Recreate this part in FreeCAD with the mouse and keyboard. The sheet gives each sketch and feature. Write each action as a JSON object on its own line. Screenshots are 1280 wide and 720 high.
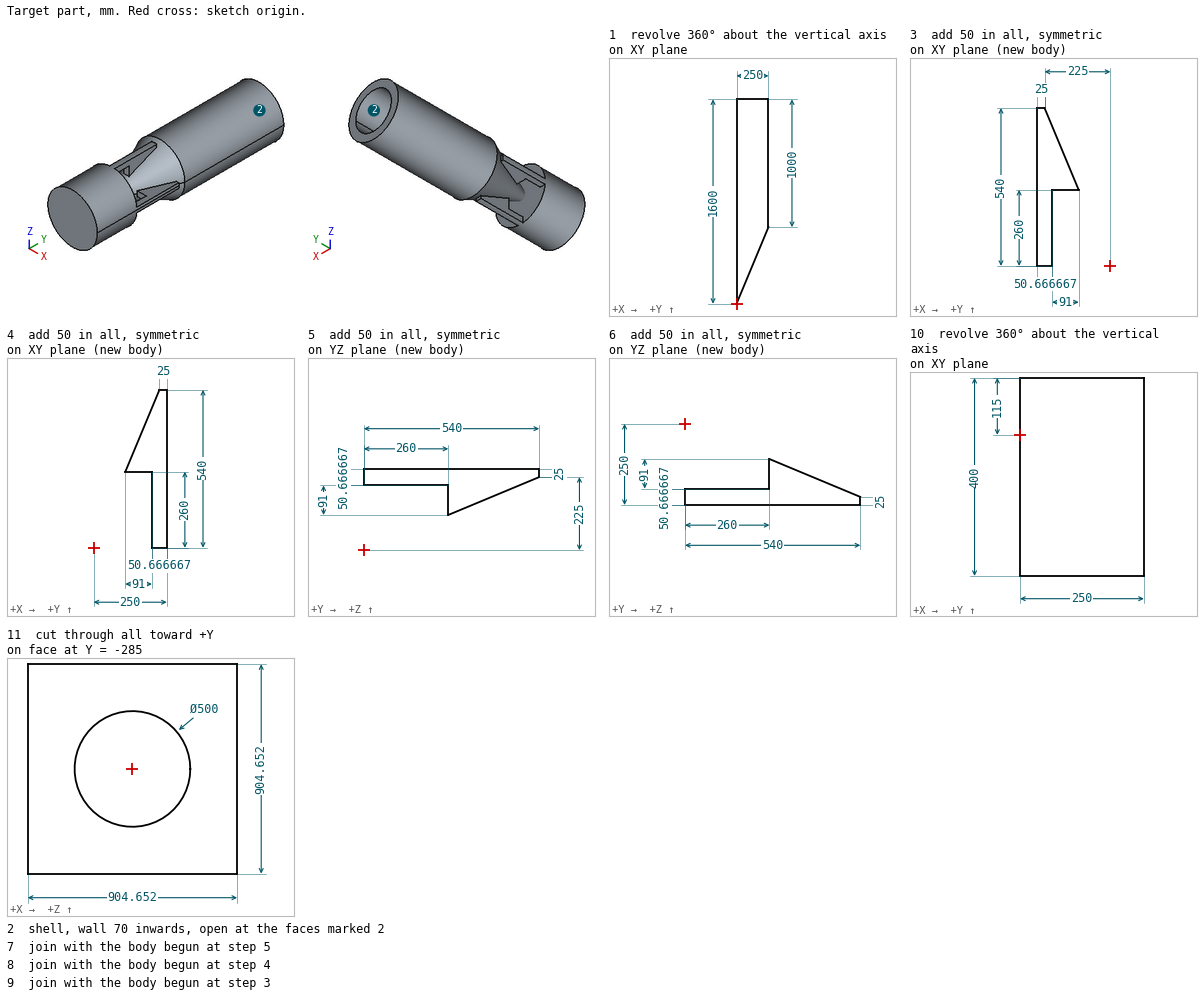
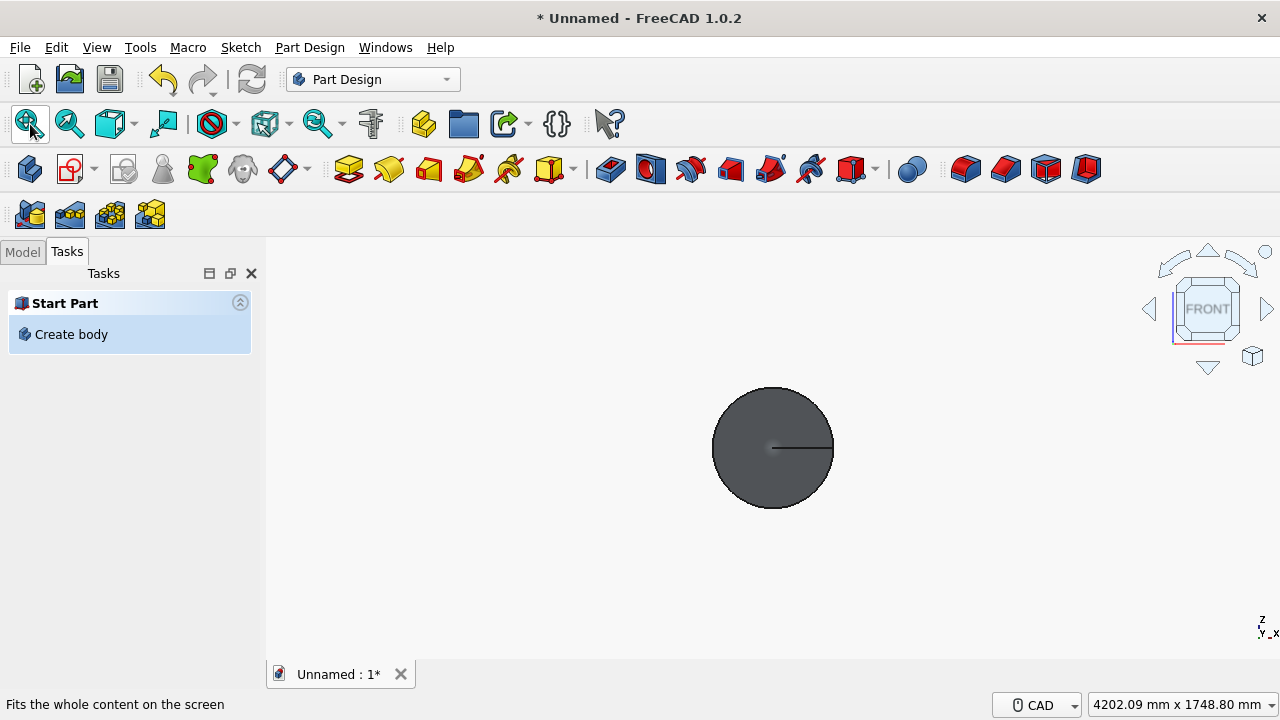
{"action": "left_click", "coordinate": [30, 124]}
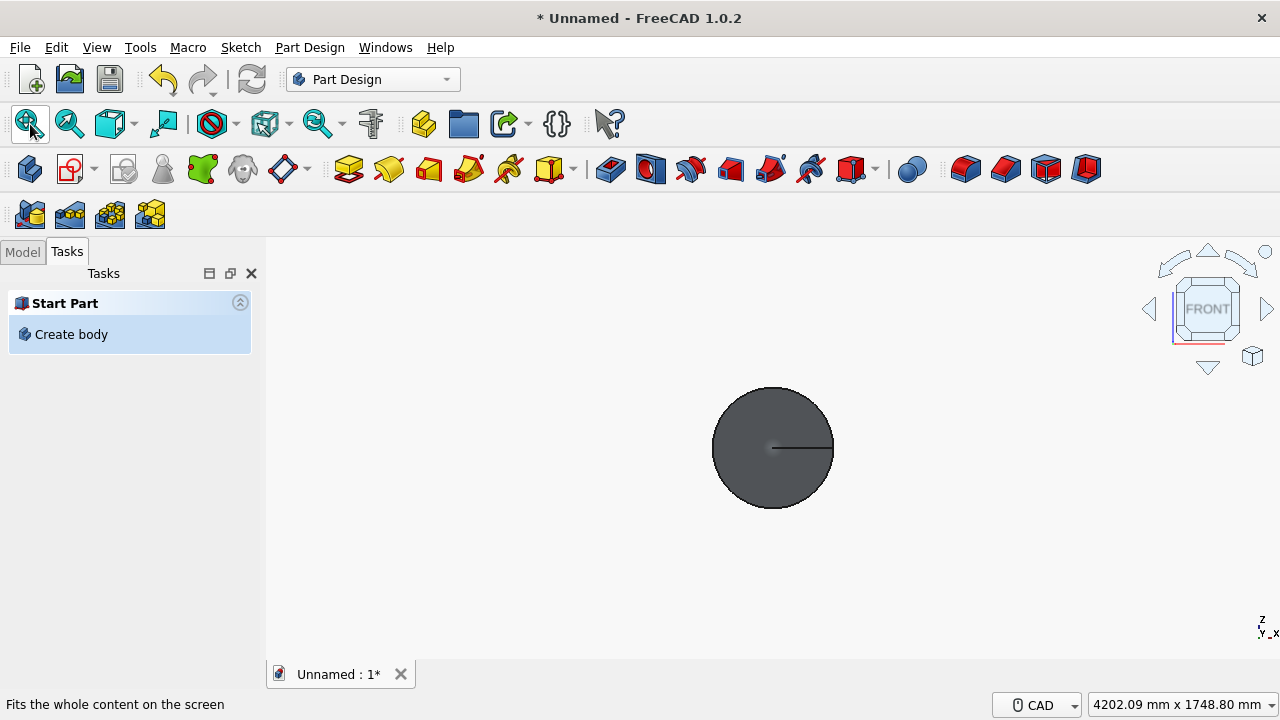
{"action": "key", "text": "3"}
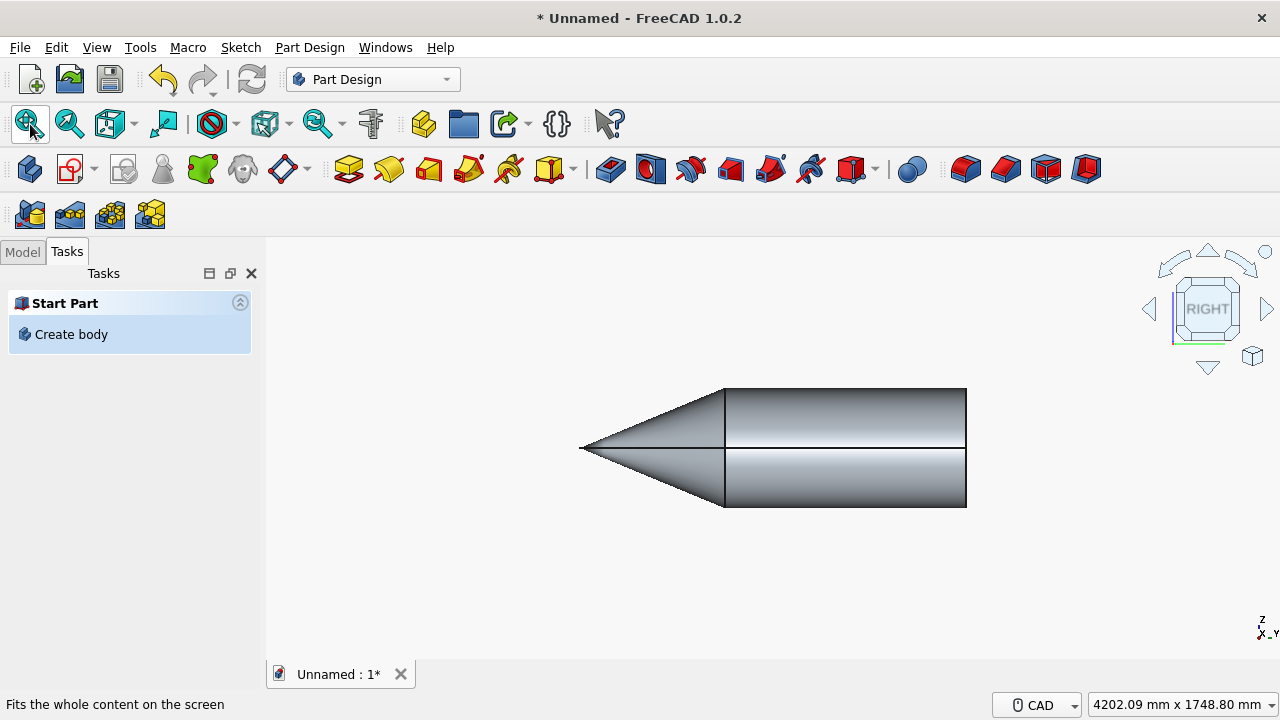
{"action": "left_click", "coordinate": [30, 124]}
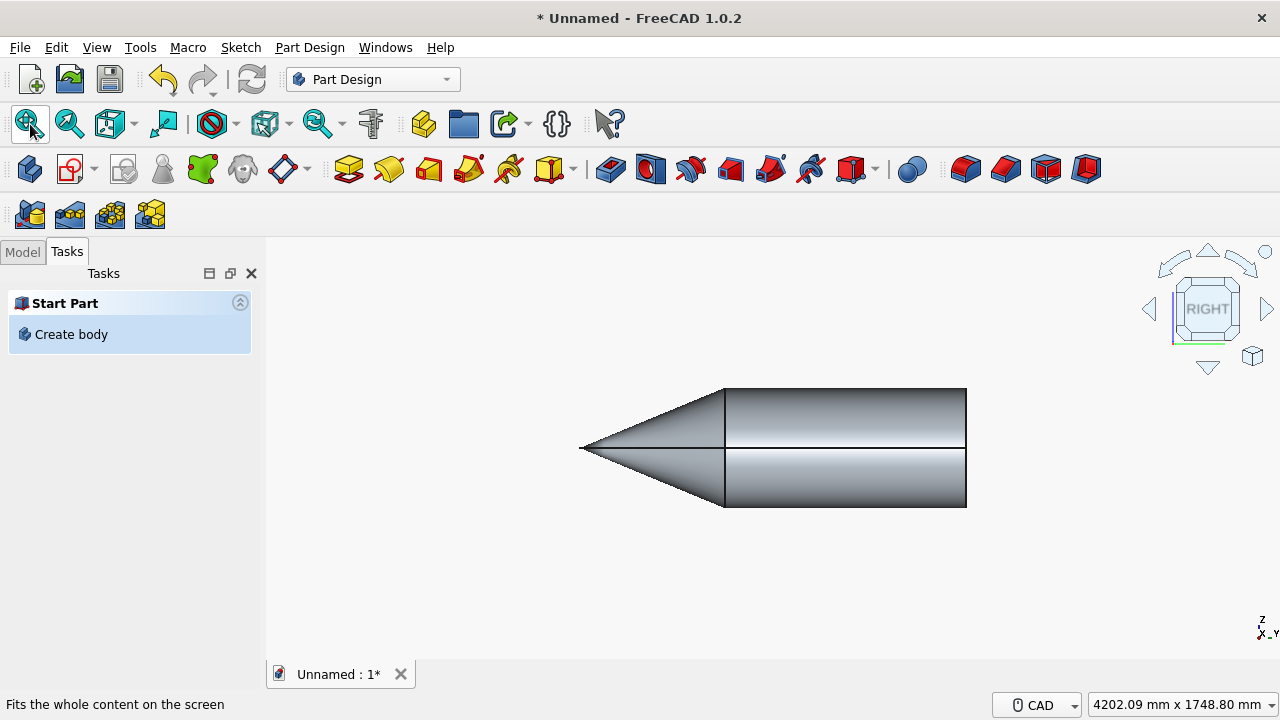
{"action": "key", "text": "5"}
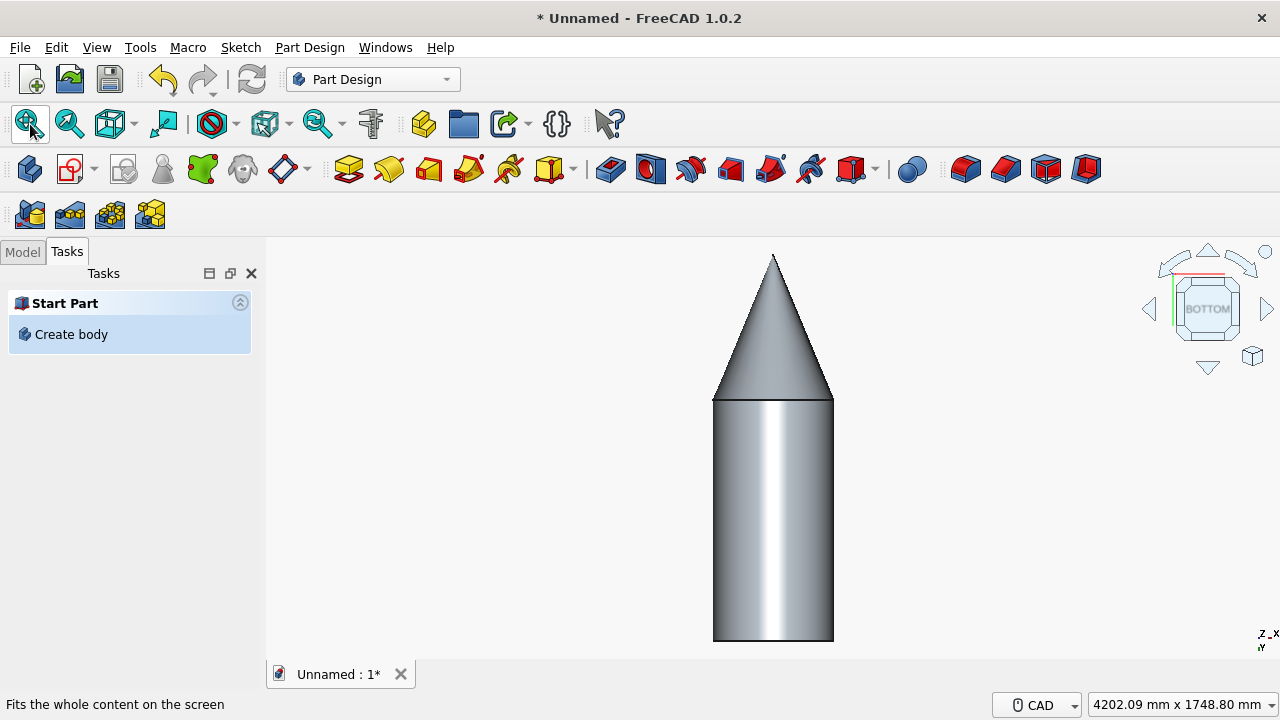
{"action": "key", "text": "4"}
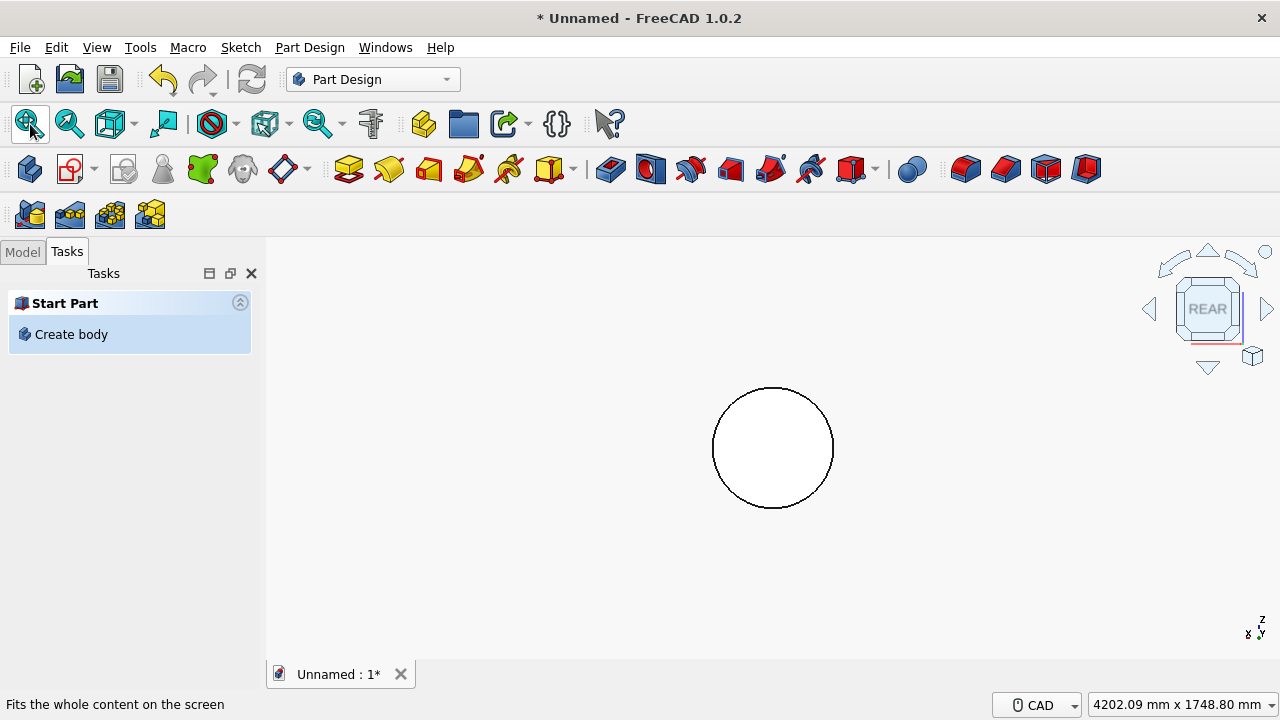
{"action": "left_click", "coordinate": [30, 124]}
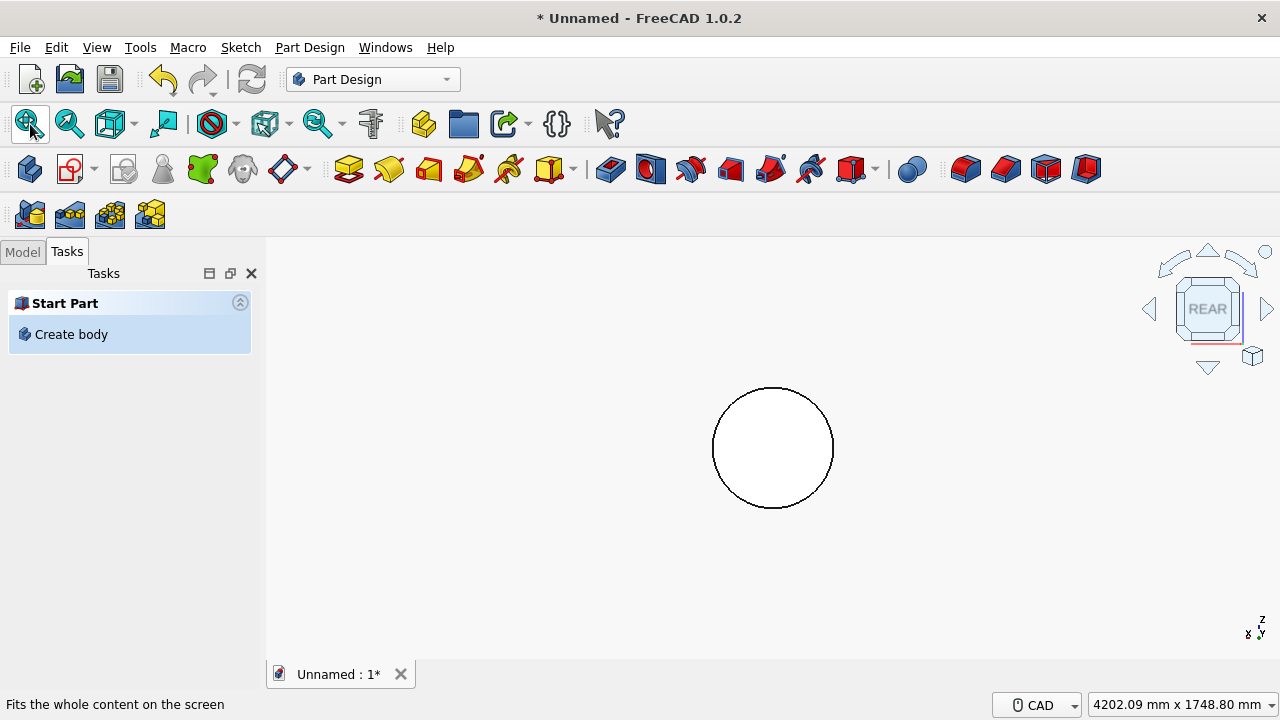
{"action": "left_click", "coordinate": [773, 447]}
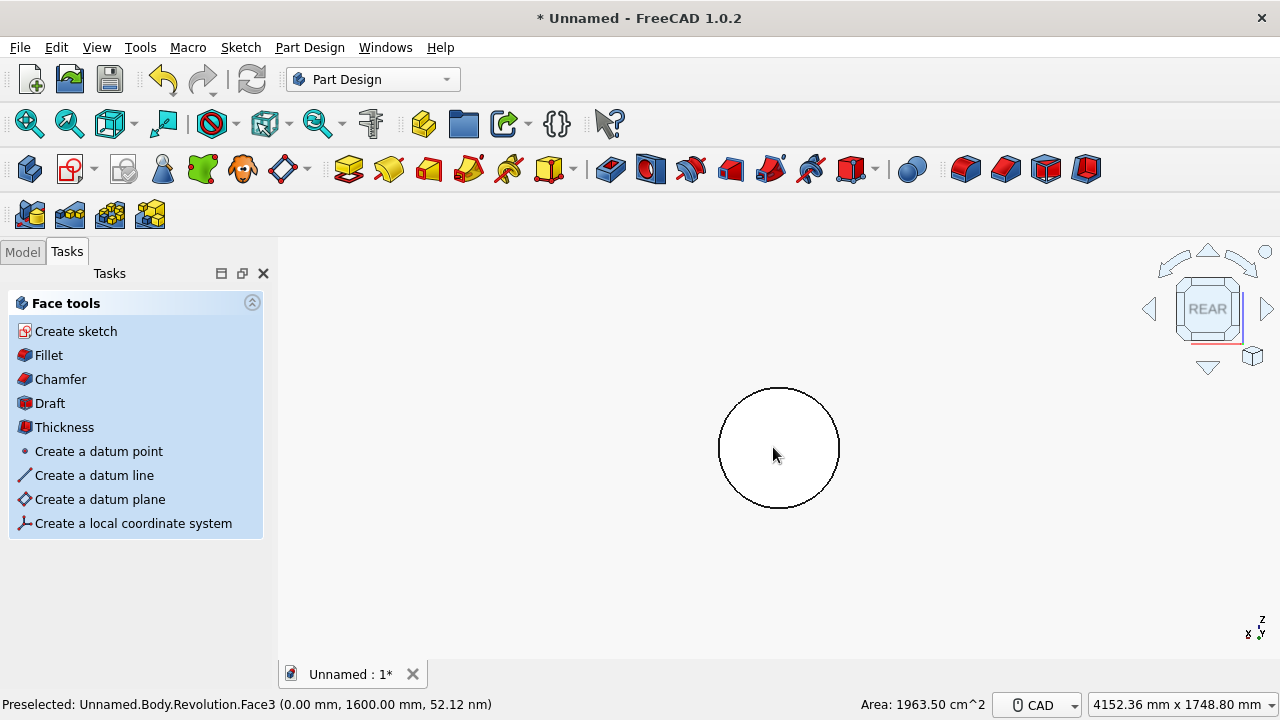
{"action": "left_click", "coordinate": [1086, 170]}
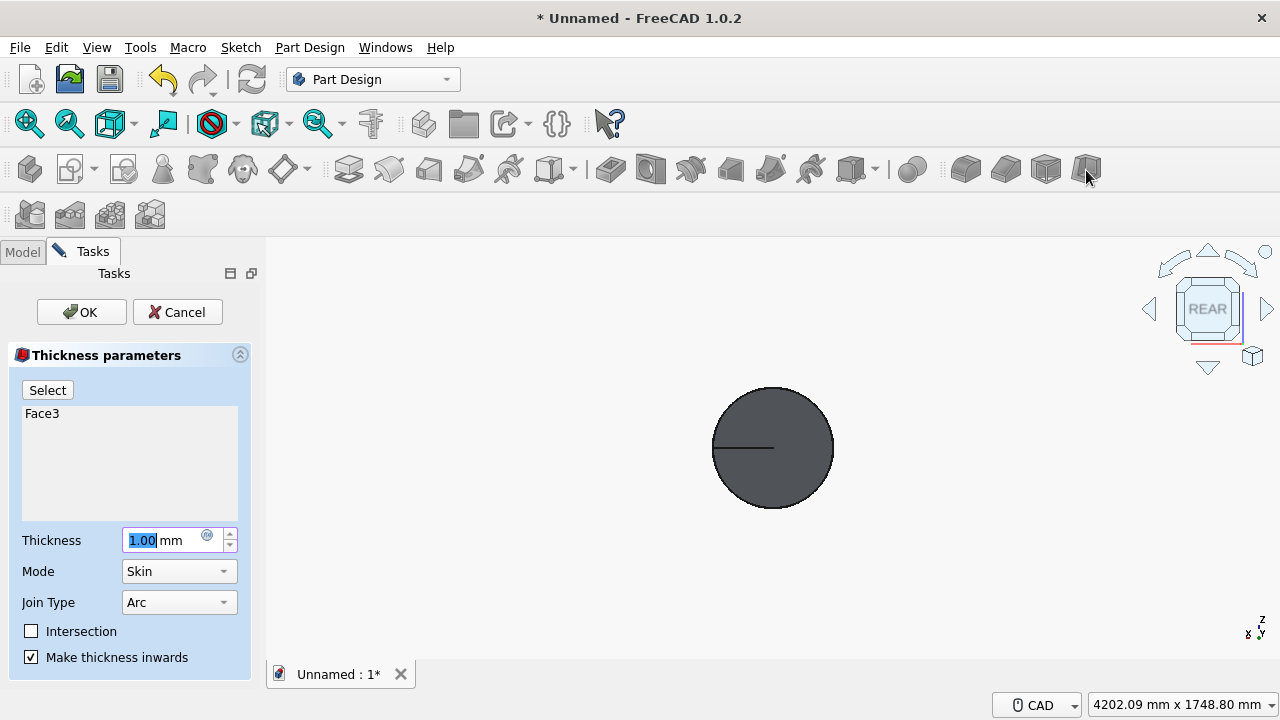
{"action": "type", "text": "70"}
{"action": "key", "text": "Tab"}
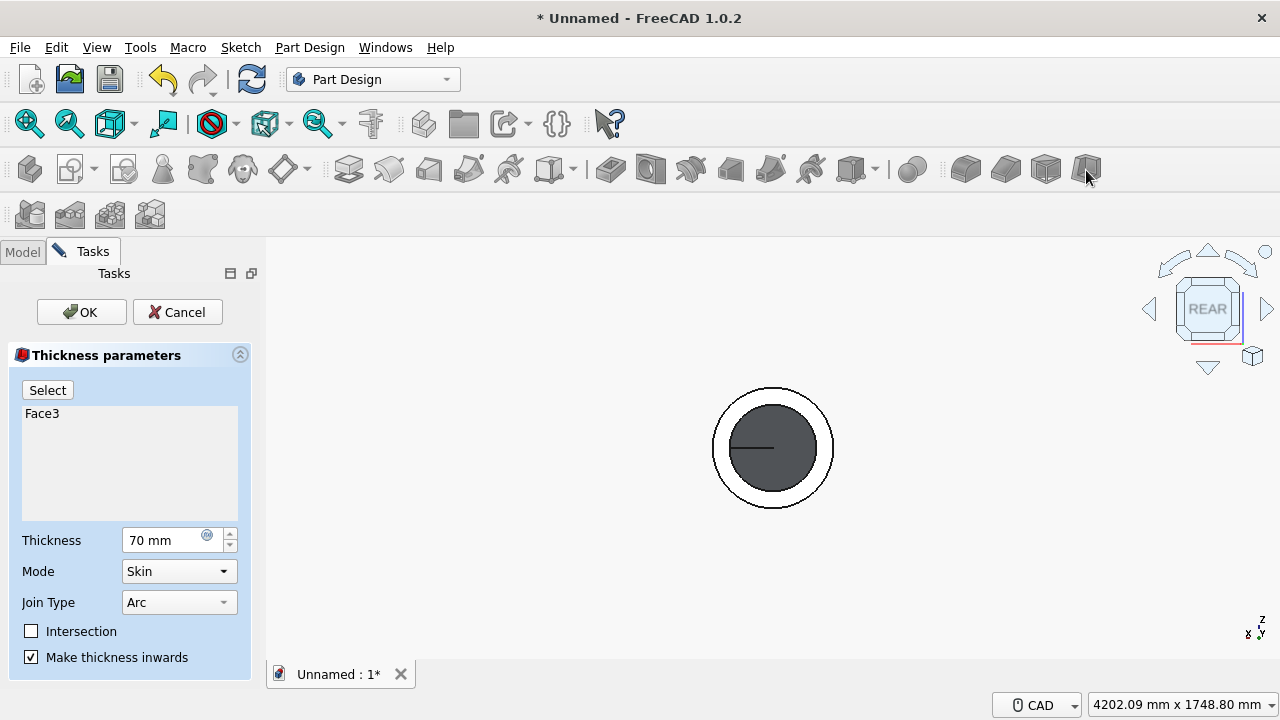
{"action": "left_click", "coordinate": [180, 602]}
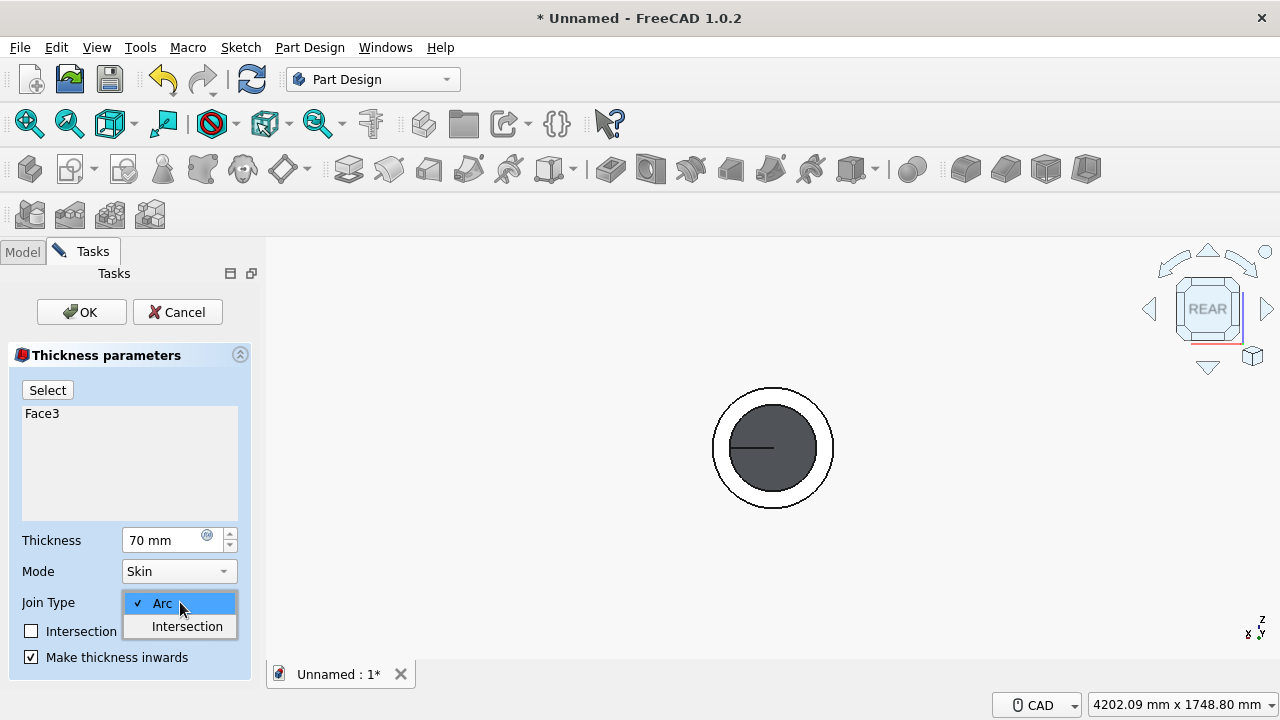
{"action": "left_click", "coordinate": [179, 626]}